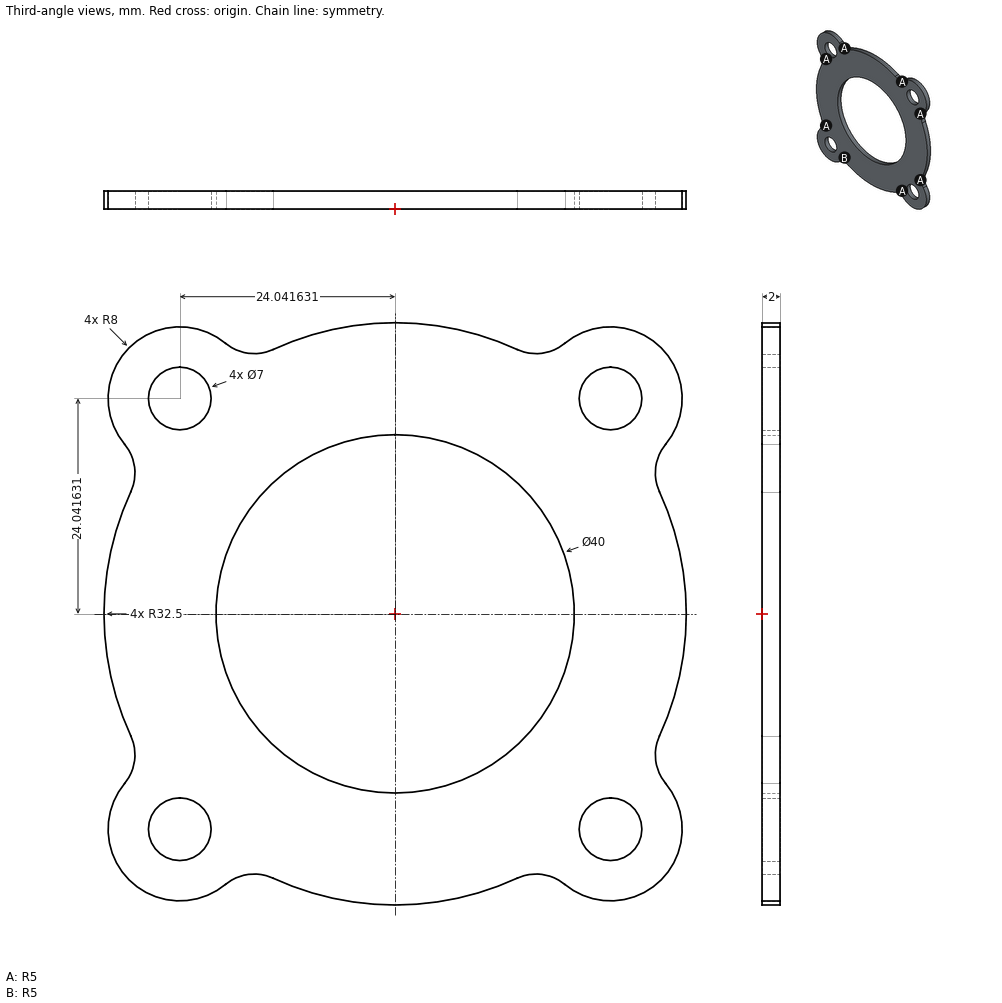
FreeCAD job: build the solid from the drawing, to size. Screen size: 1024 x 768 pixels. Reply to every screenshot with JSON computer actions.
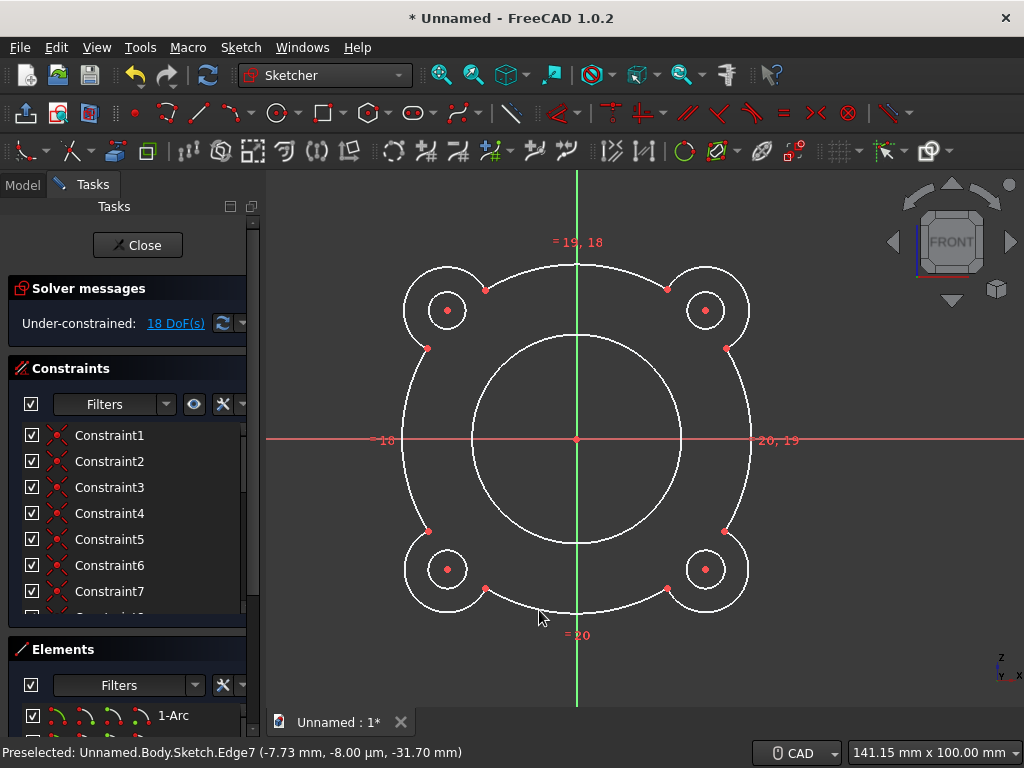
{"action": "left_click", "coordinate": [445, 267]}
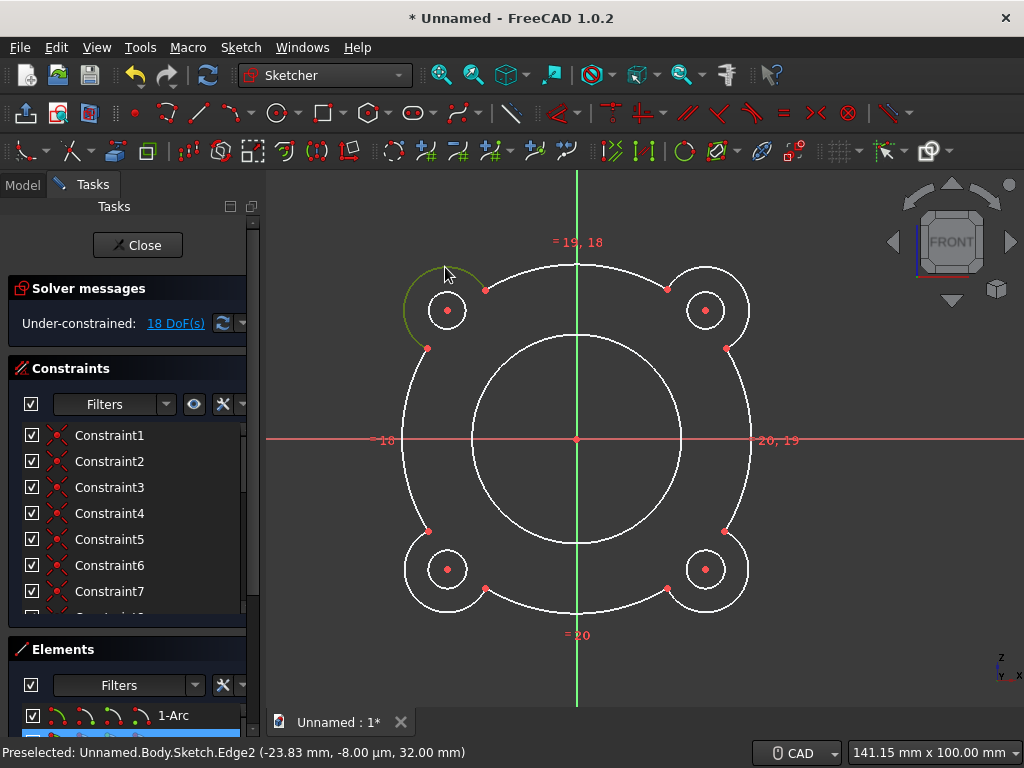
{"action": "left_click", "coordinate": [749, 309]}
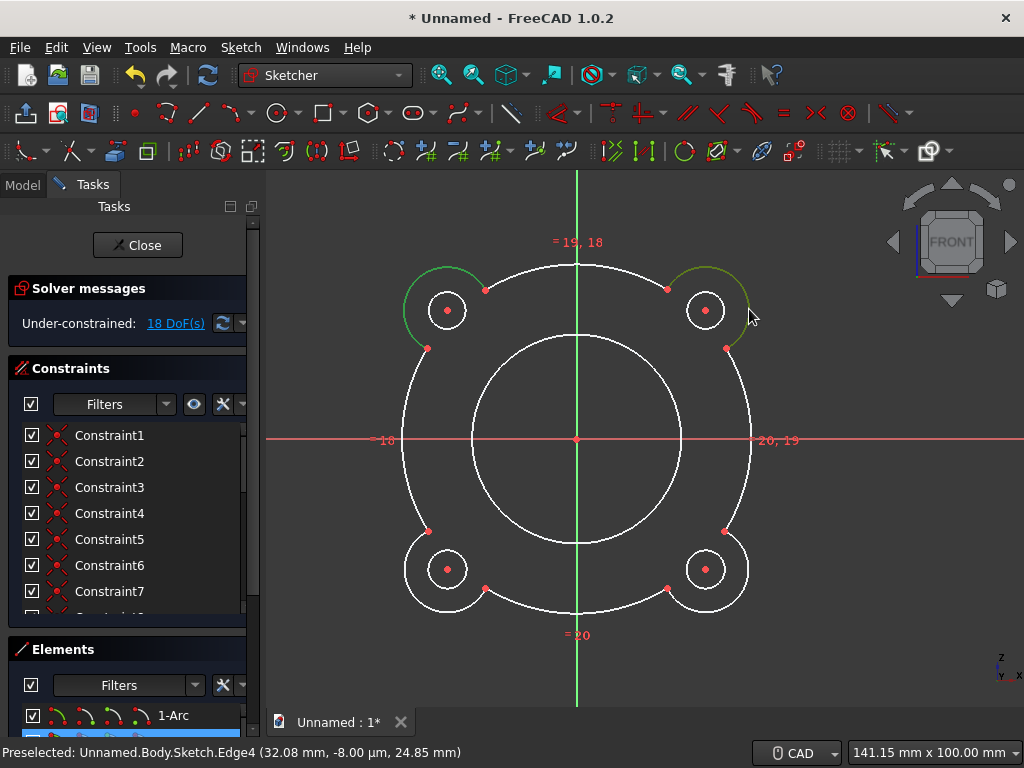
{"action": "left_click", "coordinate": [707, 612]}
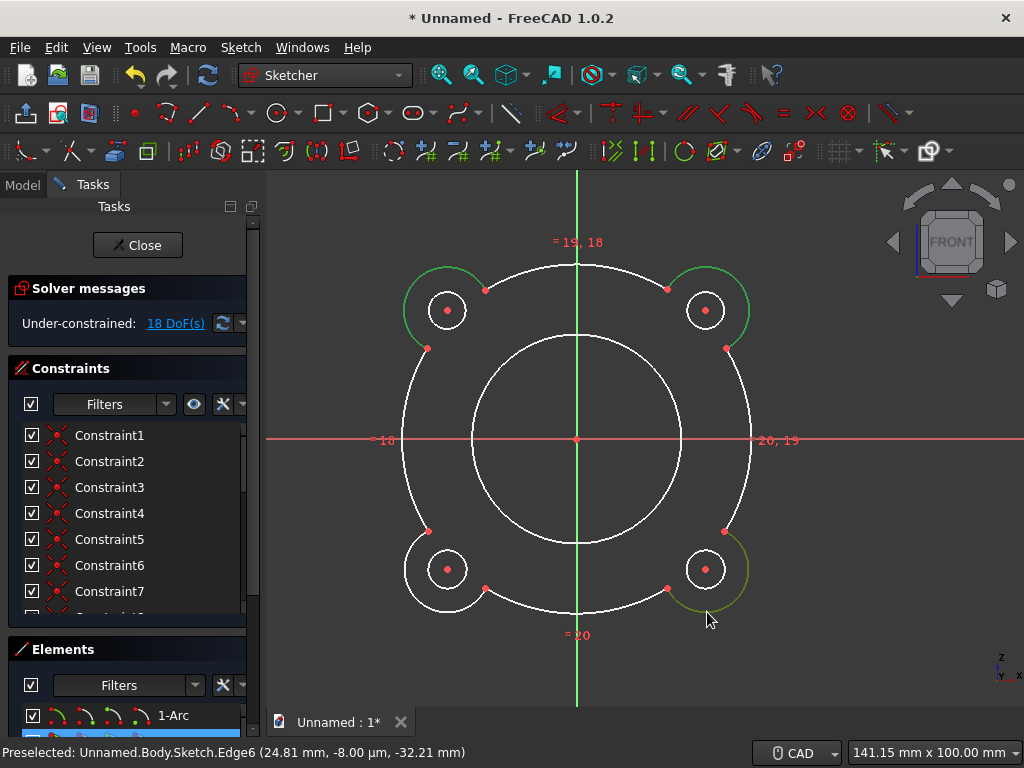
{"action": "left_click", "coordinate": [405, 571]}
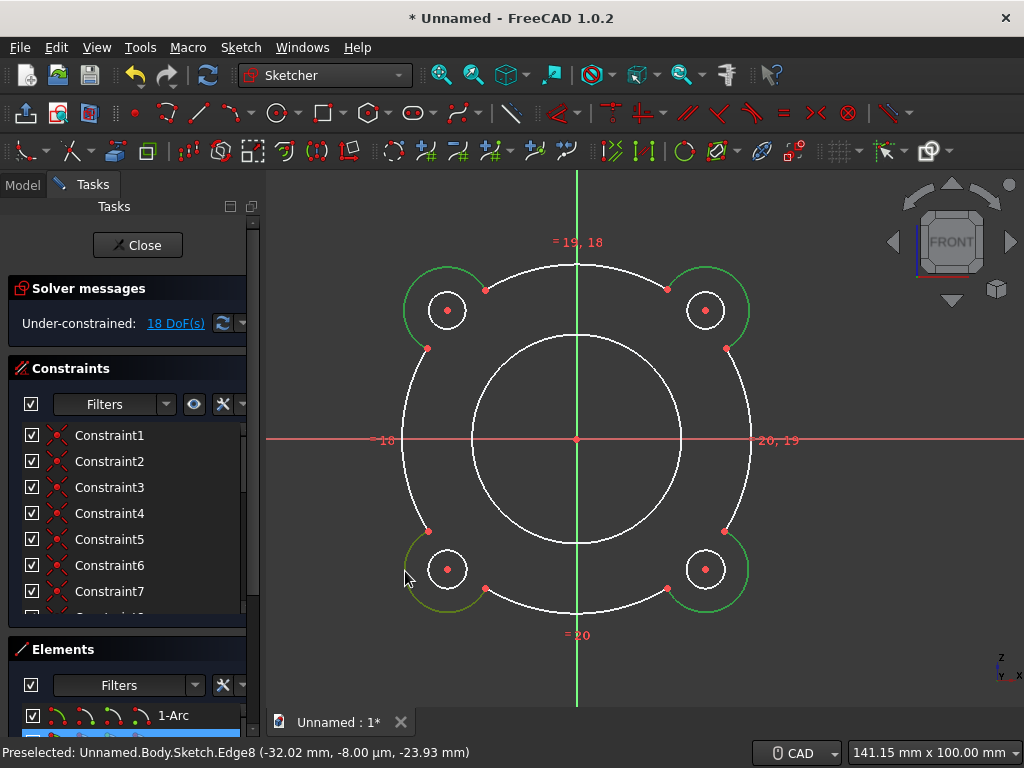
{"action": "left_click", "coordinate": [784, 114]}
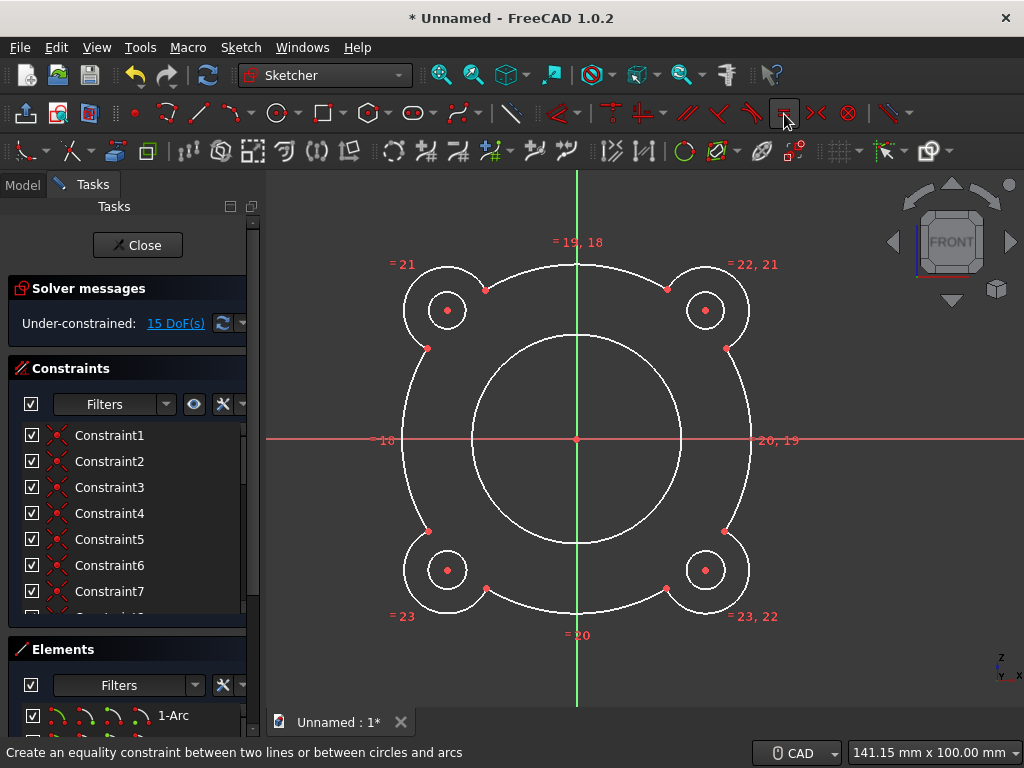
{"action": "left_click", "coordinate": [460, 297]}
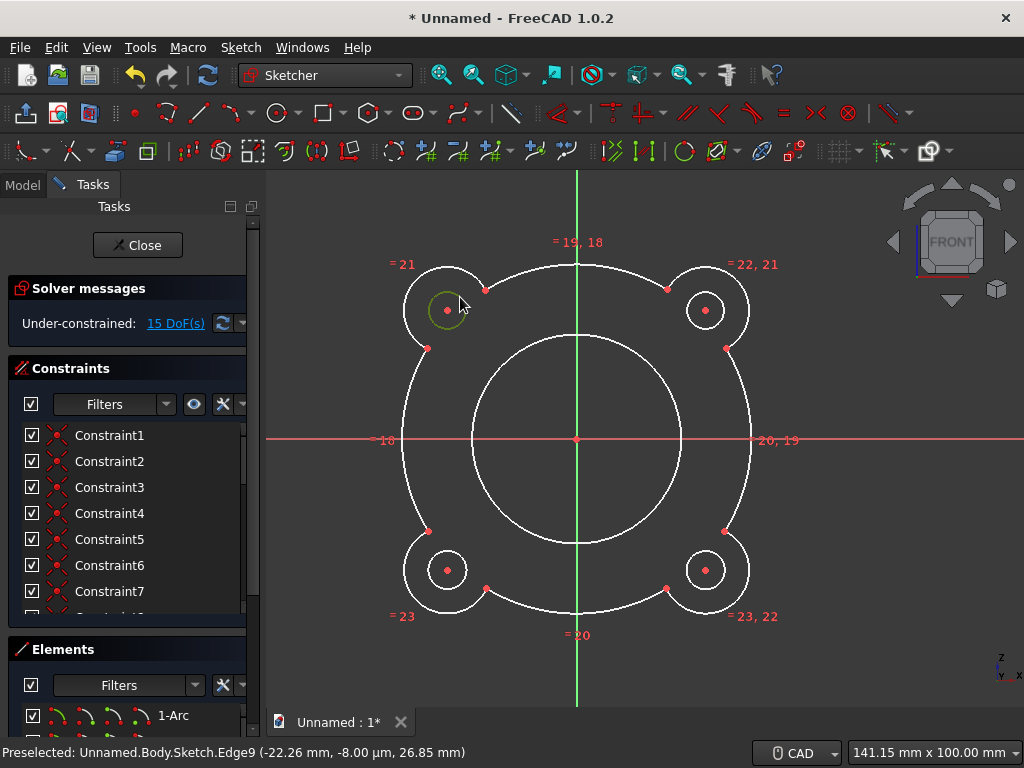
{"action": "left_click", "coordinate": [719, 297]}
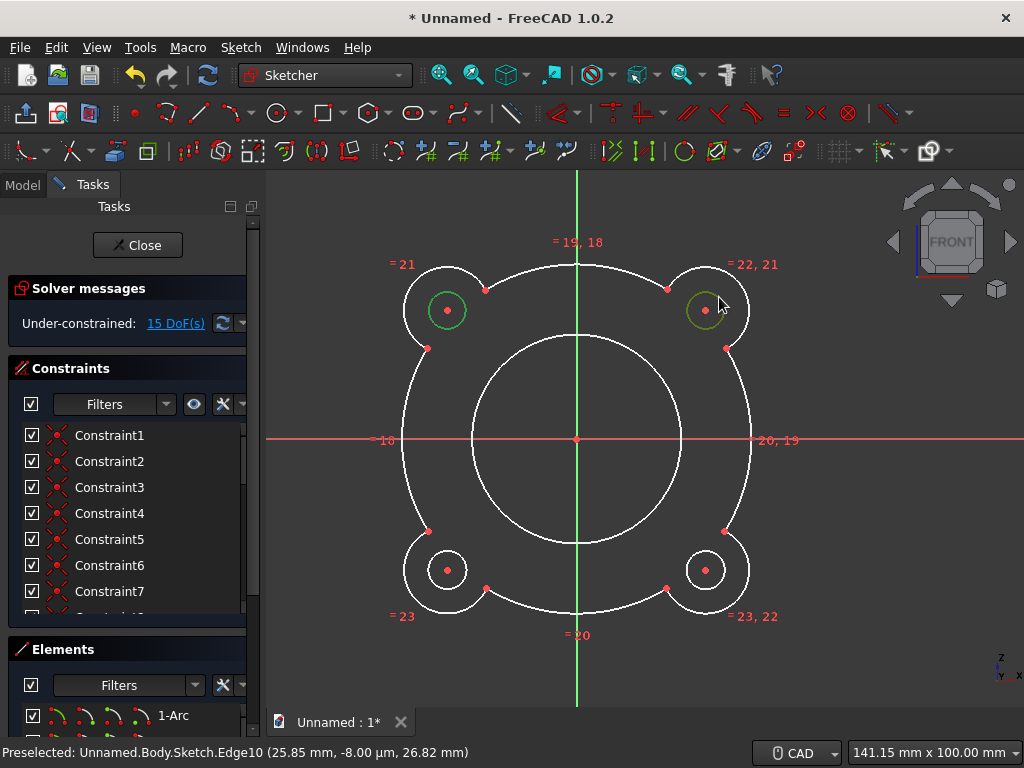
{"action": "left_click", "coordinate": [461, 556]}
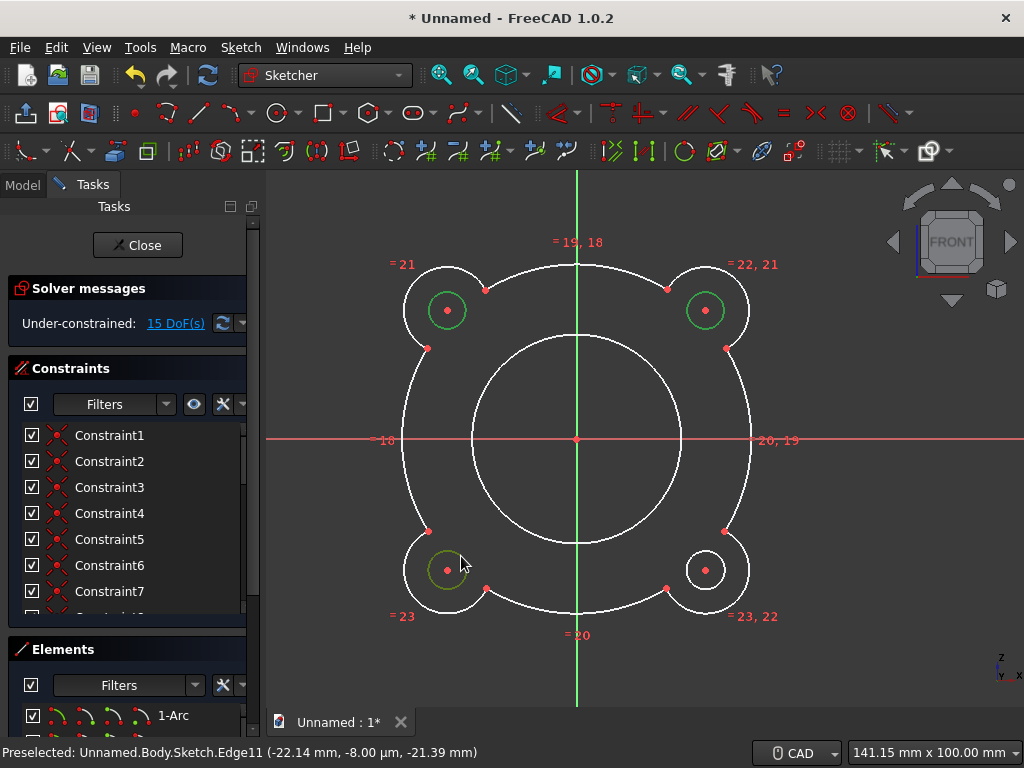
{"action": "left_click", "coordinate": [719, 557]}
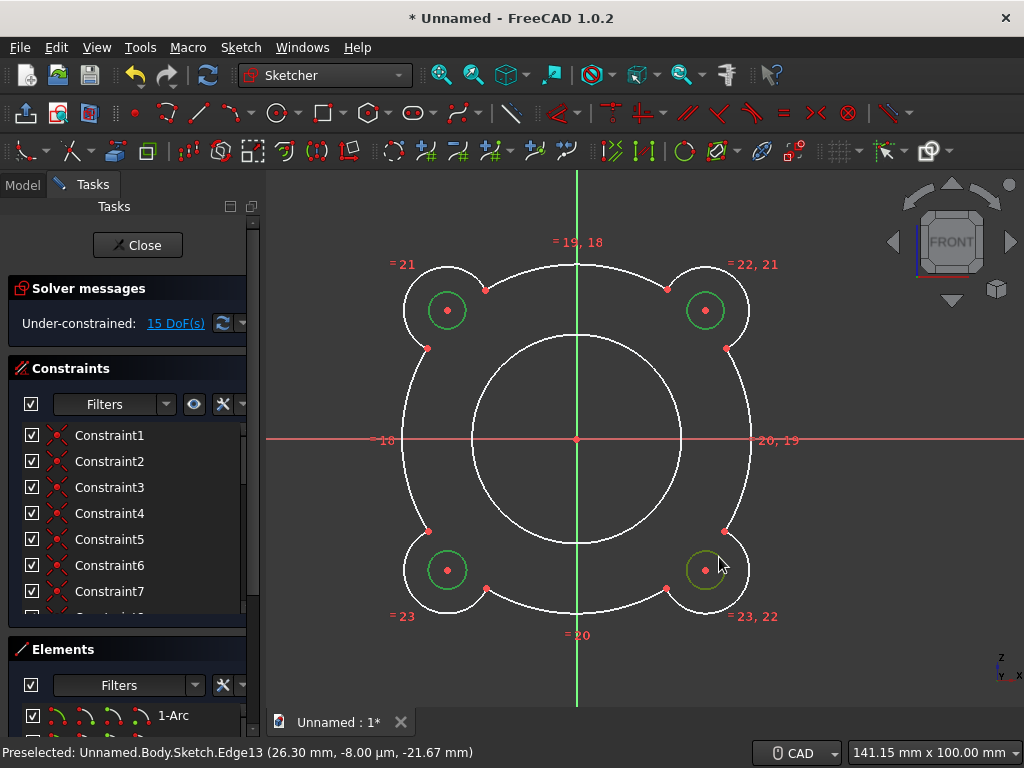
{"action": "left_click", "coordinate": [784, 114]}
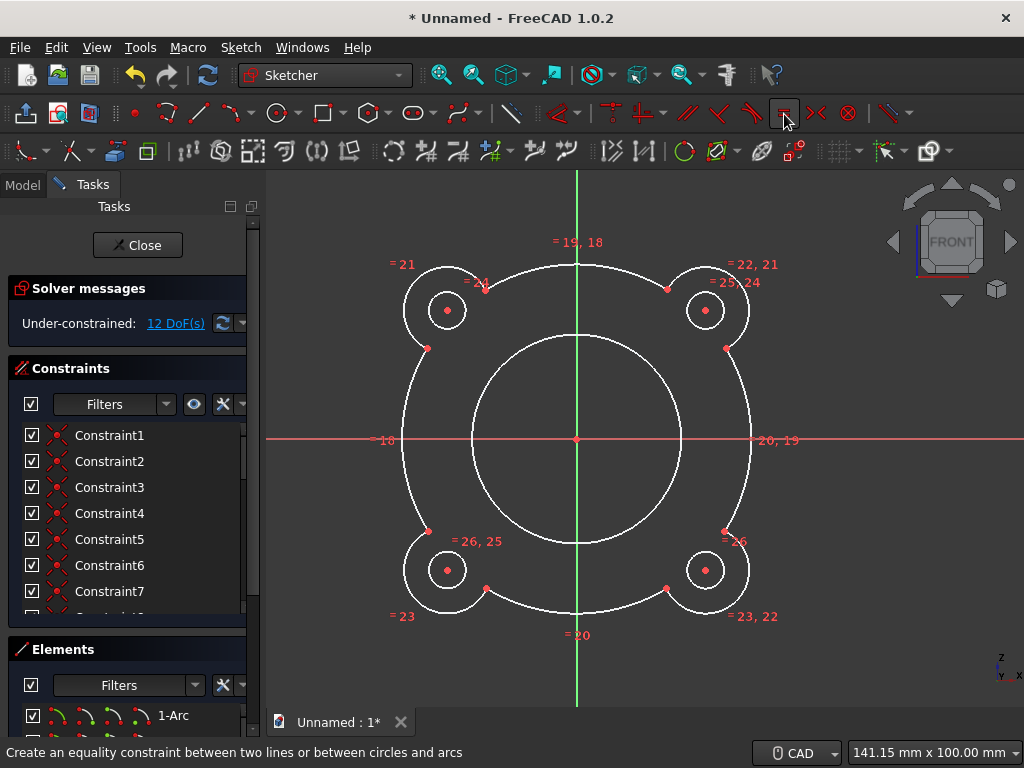
{"action": "left_click", "coordinate": [447, 310]}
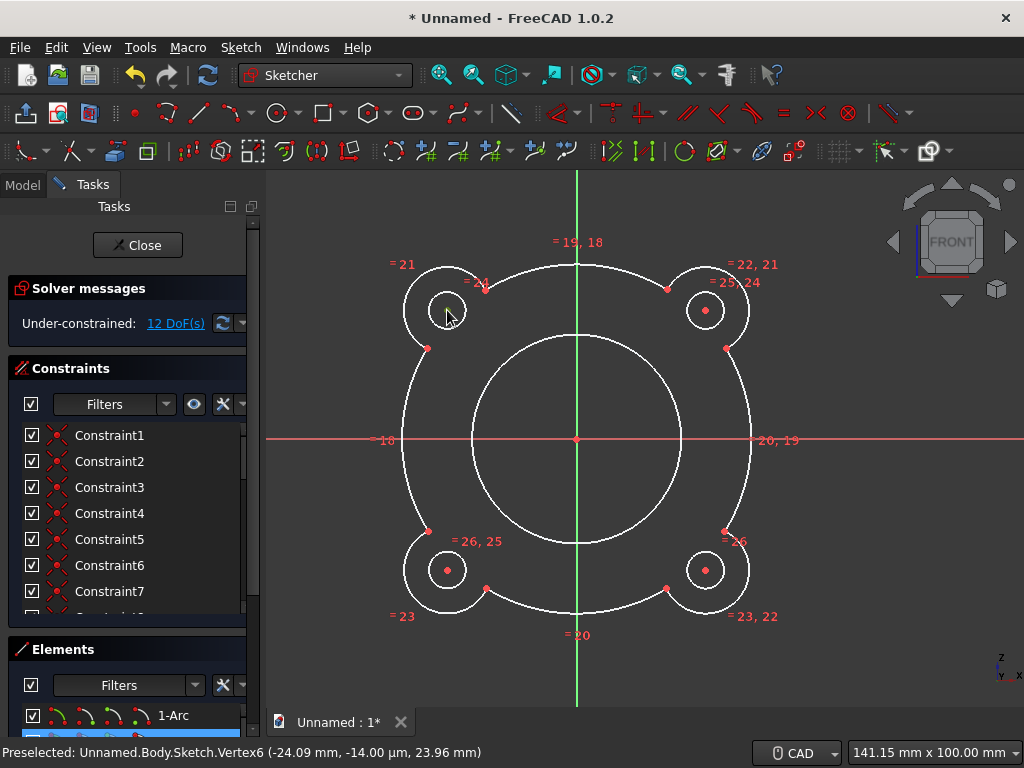
{"action": "left_click", "coordinate": [706, 311]}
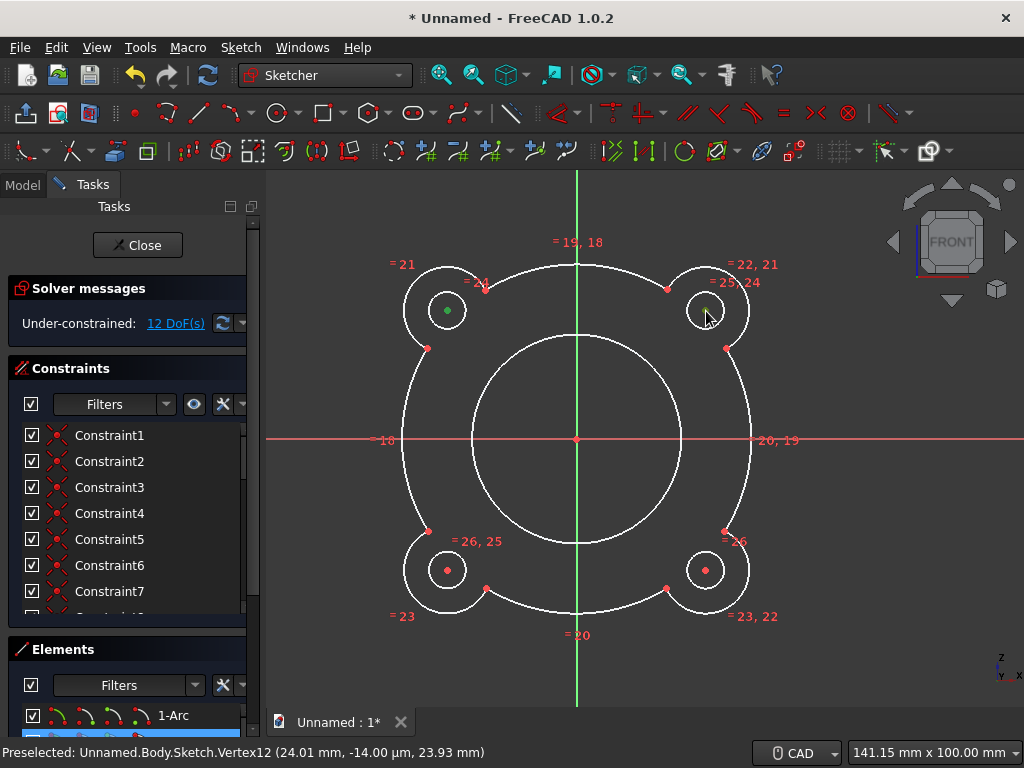
{"action": "left_click", "coordinate": [577, 645]}